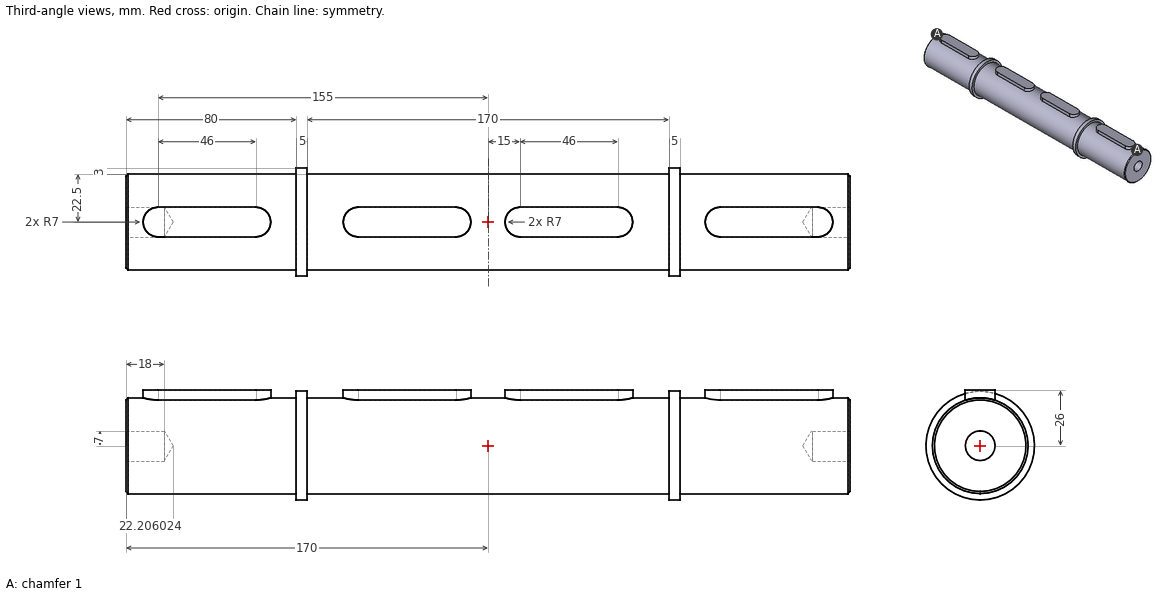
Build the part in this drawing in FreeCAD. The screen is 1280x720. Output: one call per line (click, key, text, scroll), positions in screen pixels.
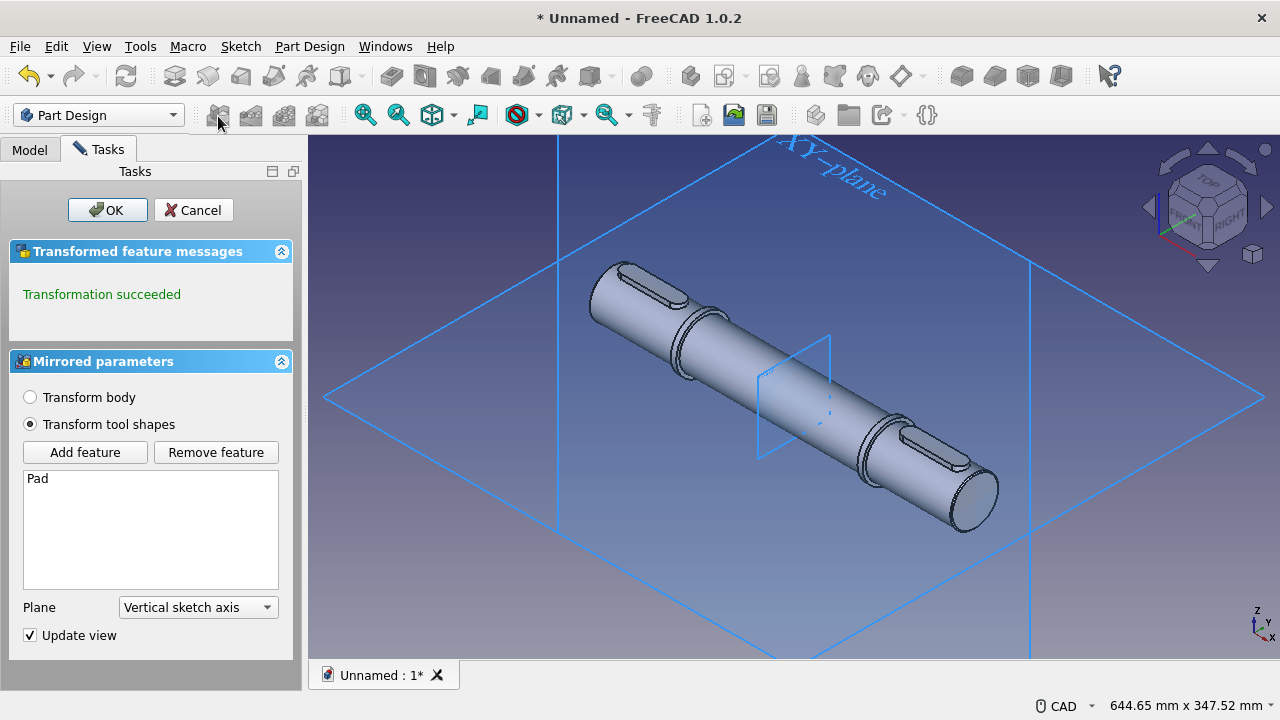
click(199, 608)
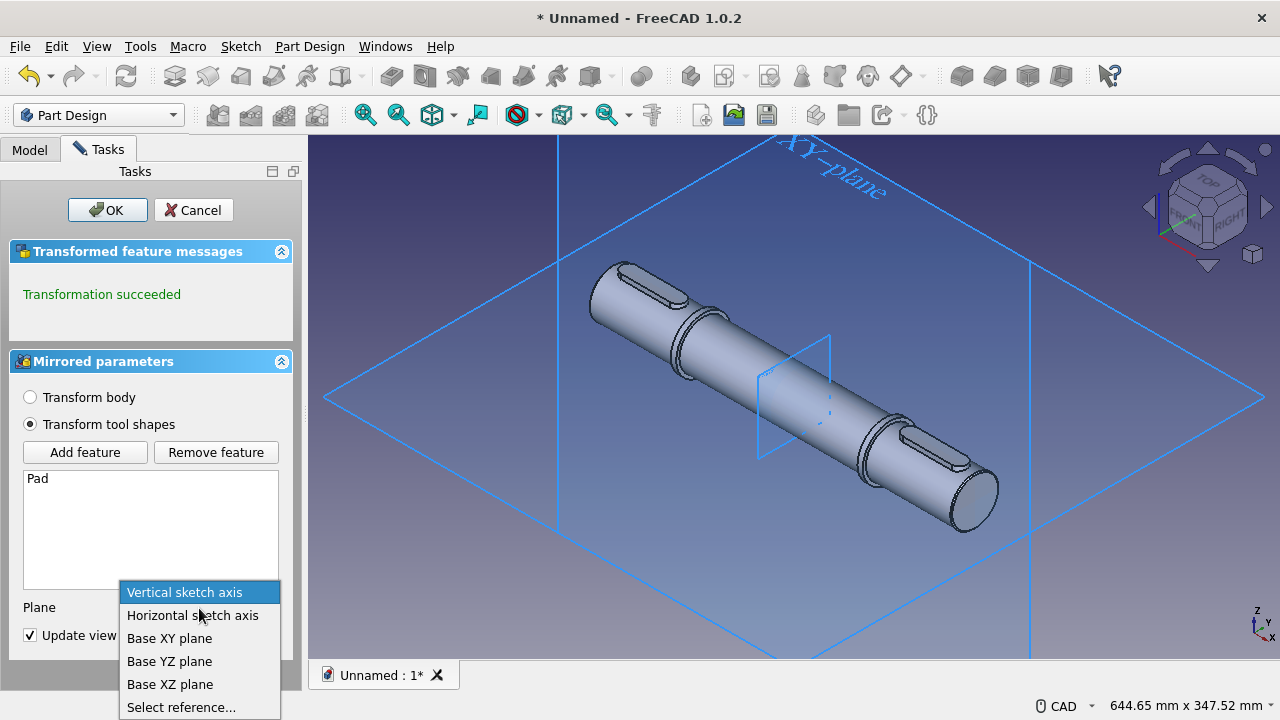
click(198, 662)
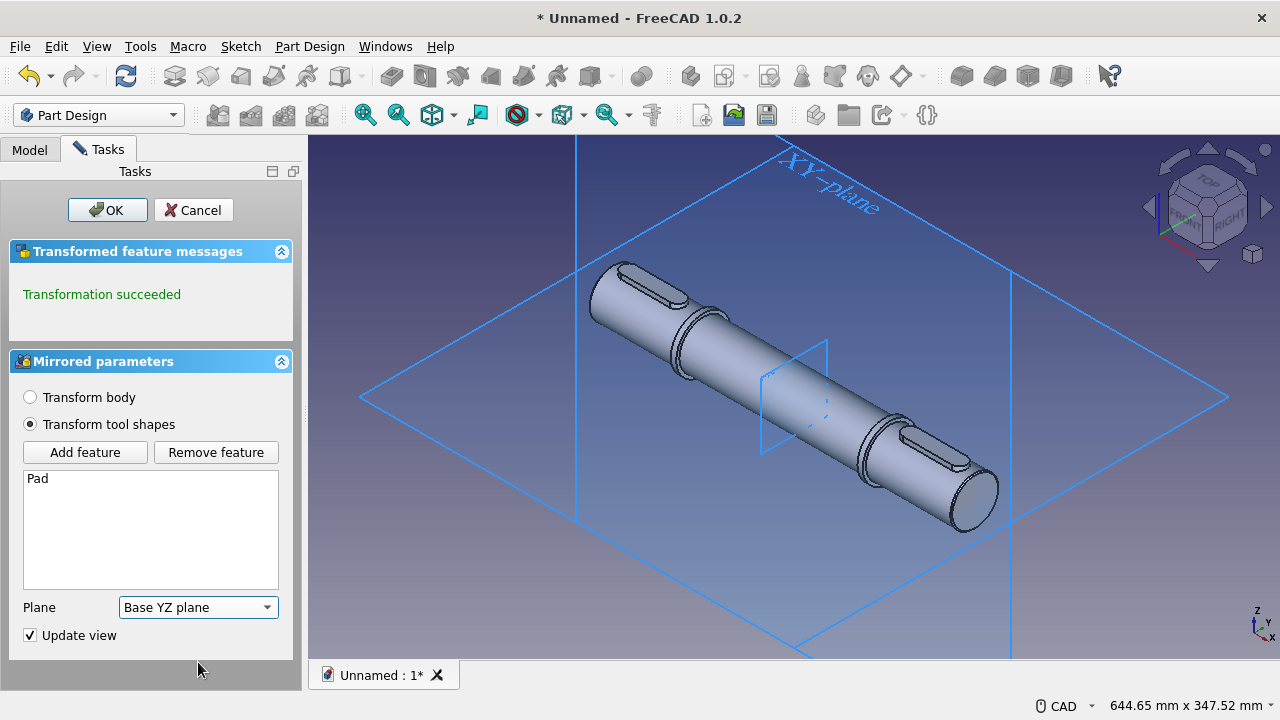
click(108, 210)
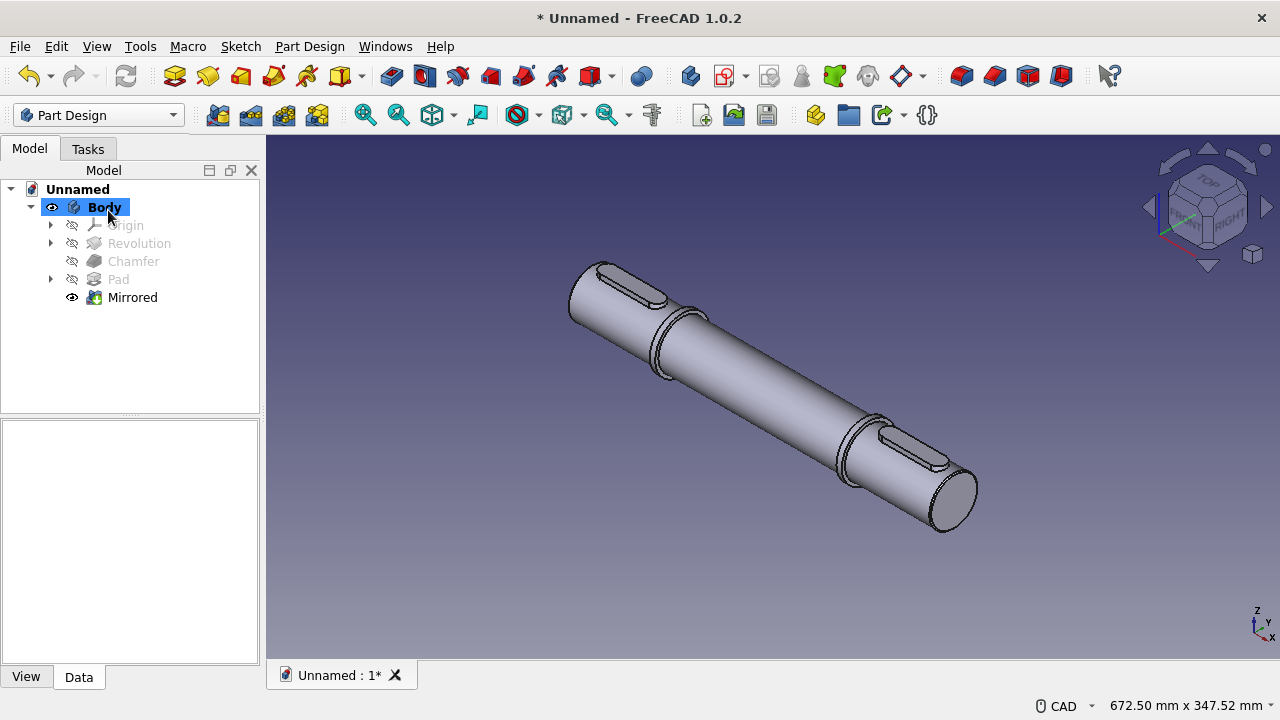
click(724, 76)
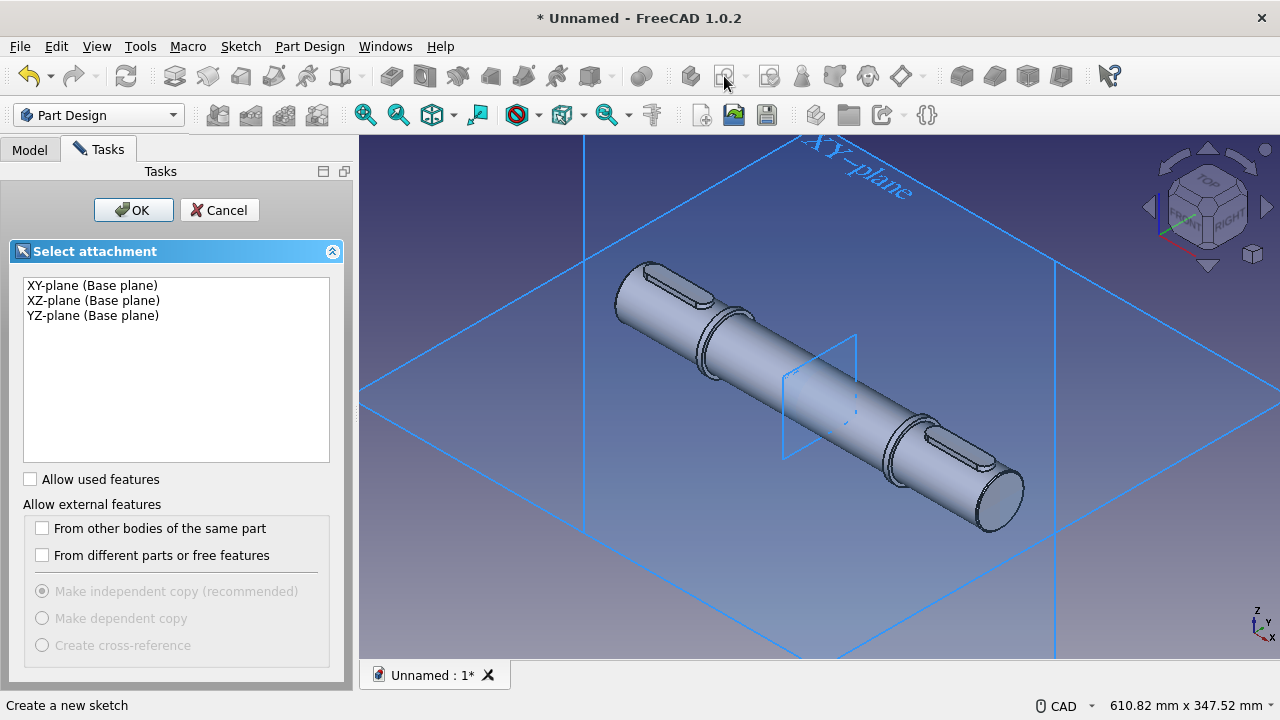
click(84, 300)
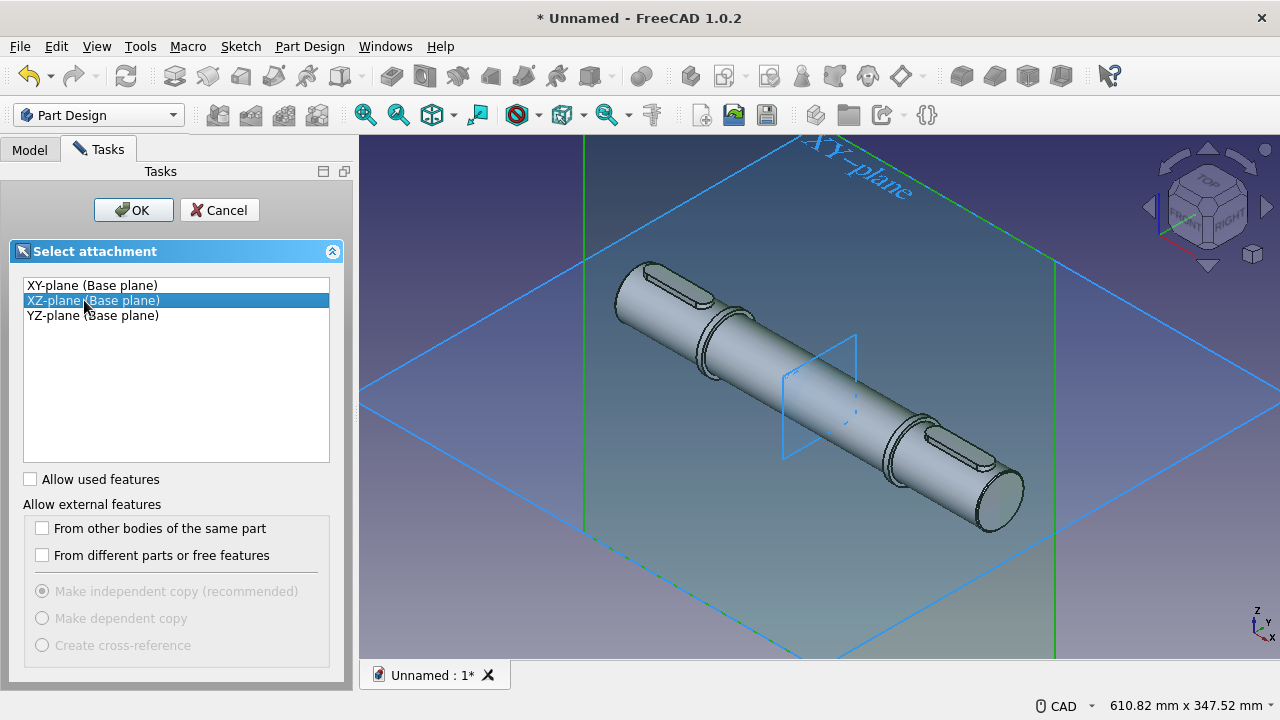
click(134, 210)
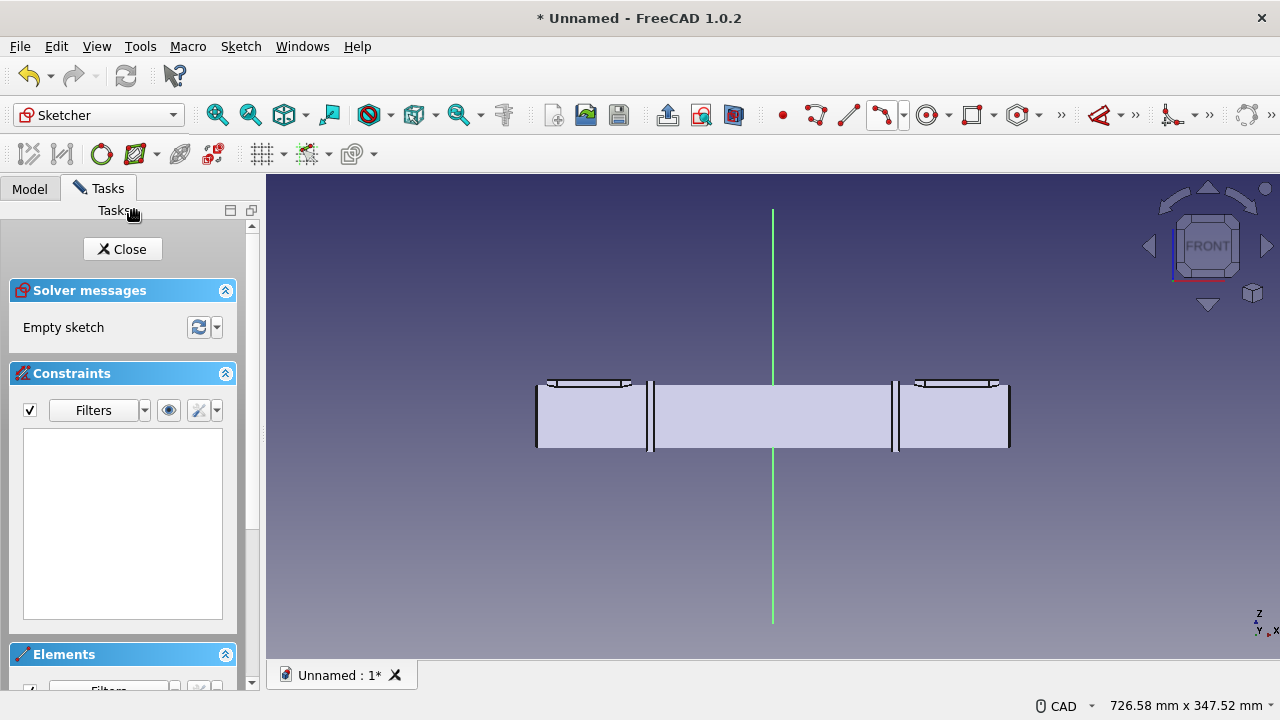
key(q)
key(s)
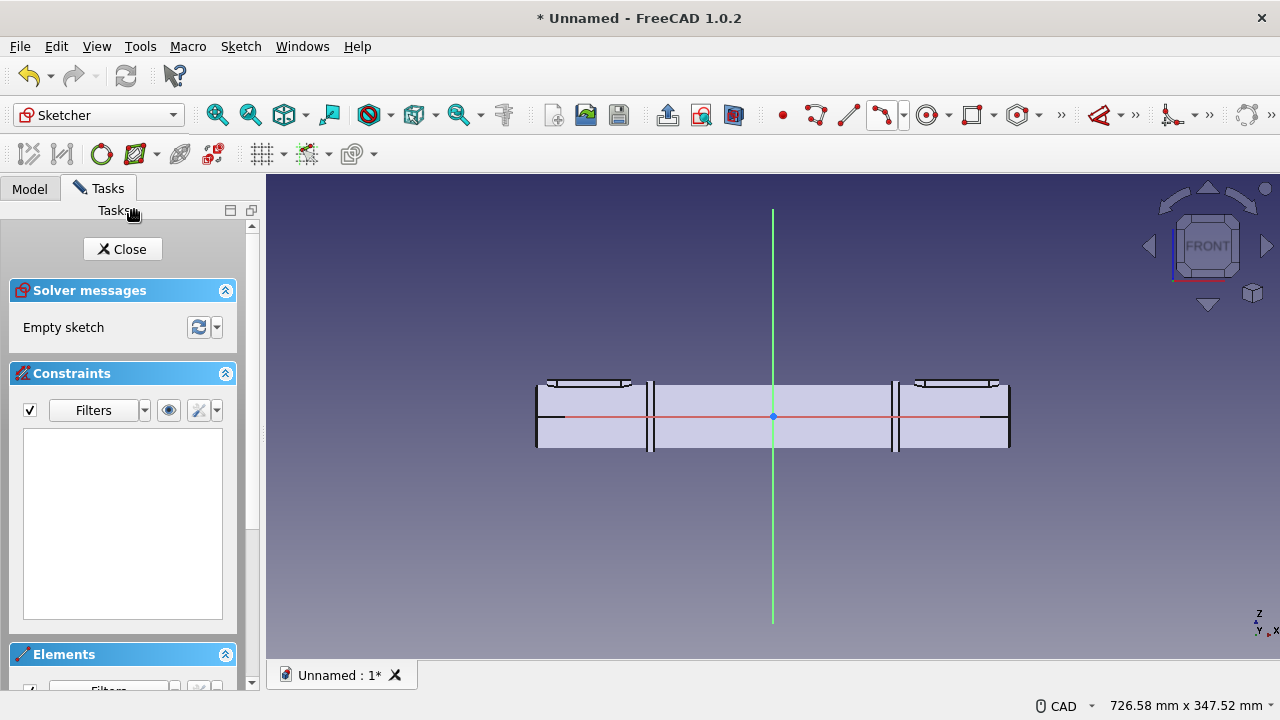
scroll(543, 411, up, 15)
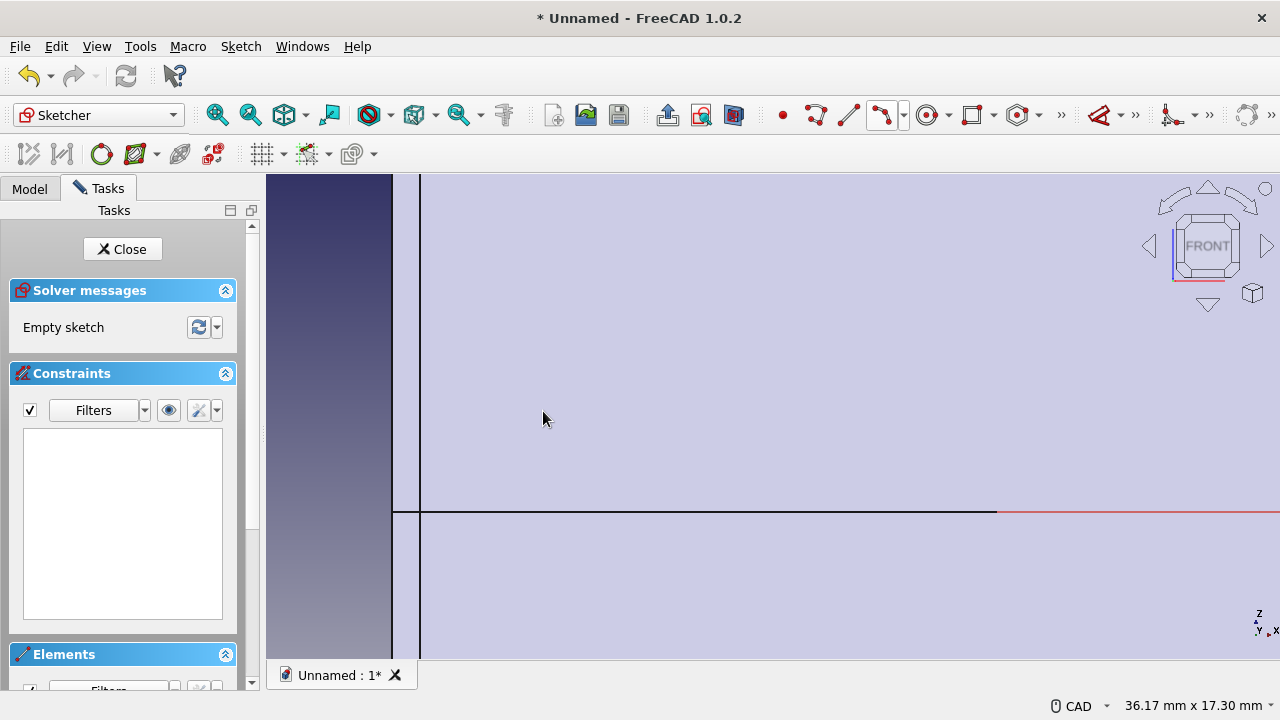
click(816, 116)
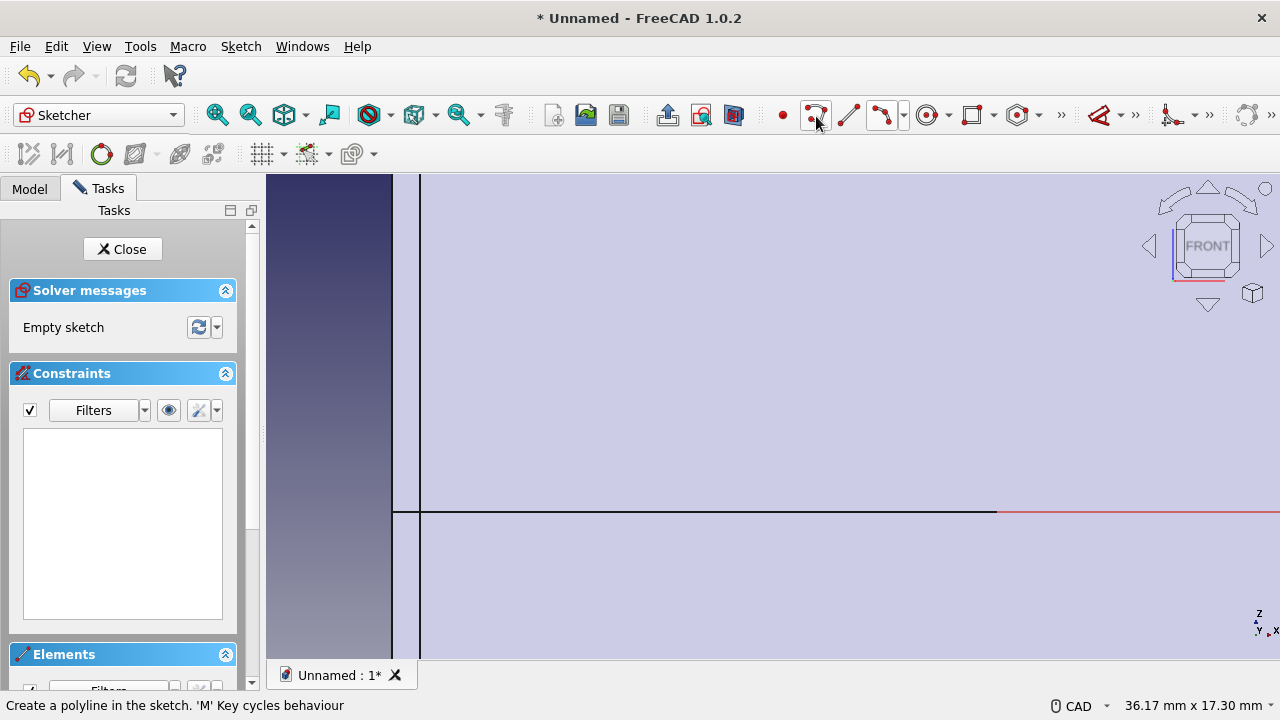
click(1015, 512)
click(392, 503)
click(392, 316)
click(897, 316)
click(1015, 512)
key(Escape)
key(Escape)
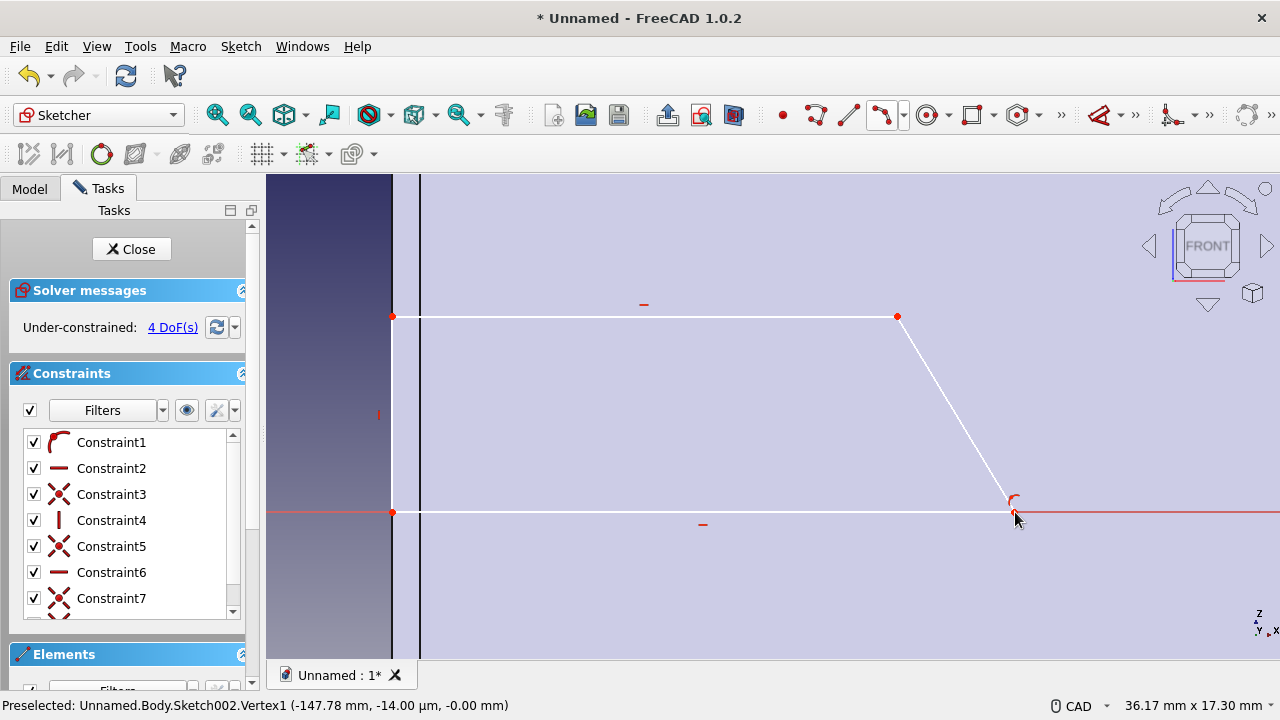
click(1098, 116)